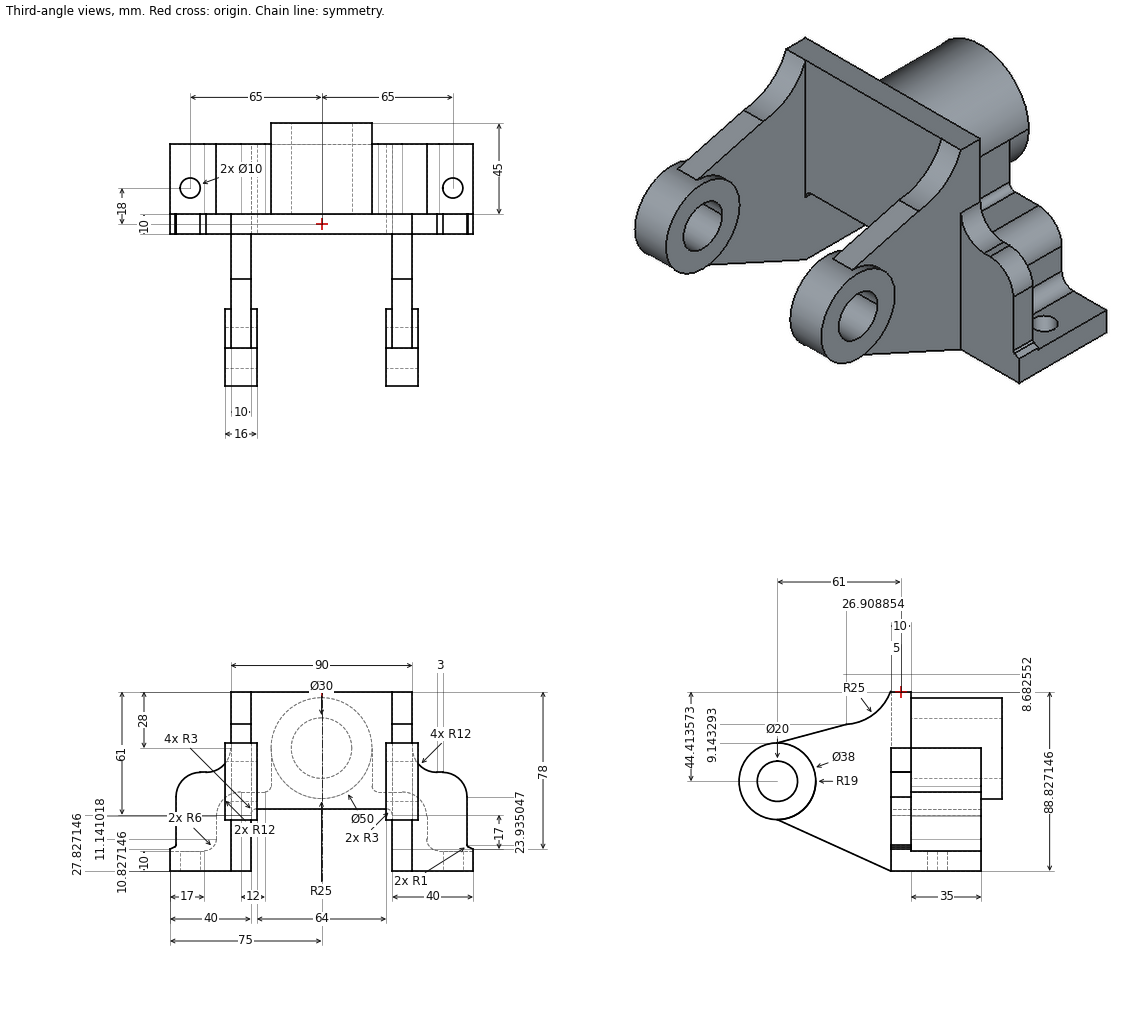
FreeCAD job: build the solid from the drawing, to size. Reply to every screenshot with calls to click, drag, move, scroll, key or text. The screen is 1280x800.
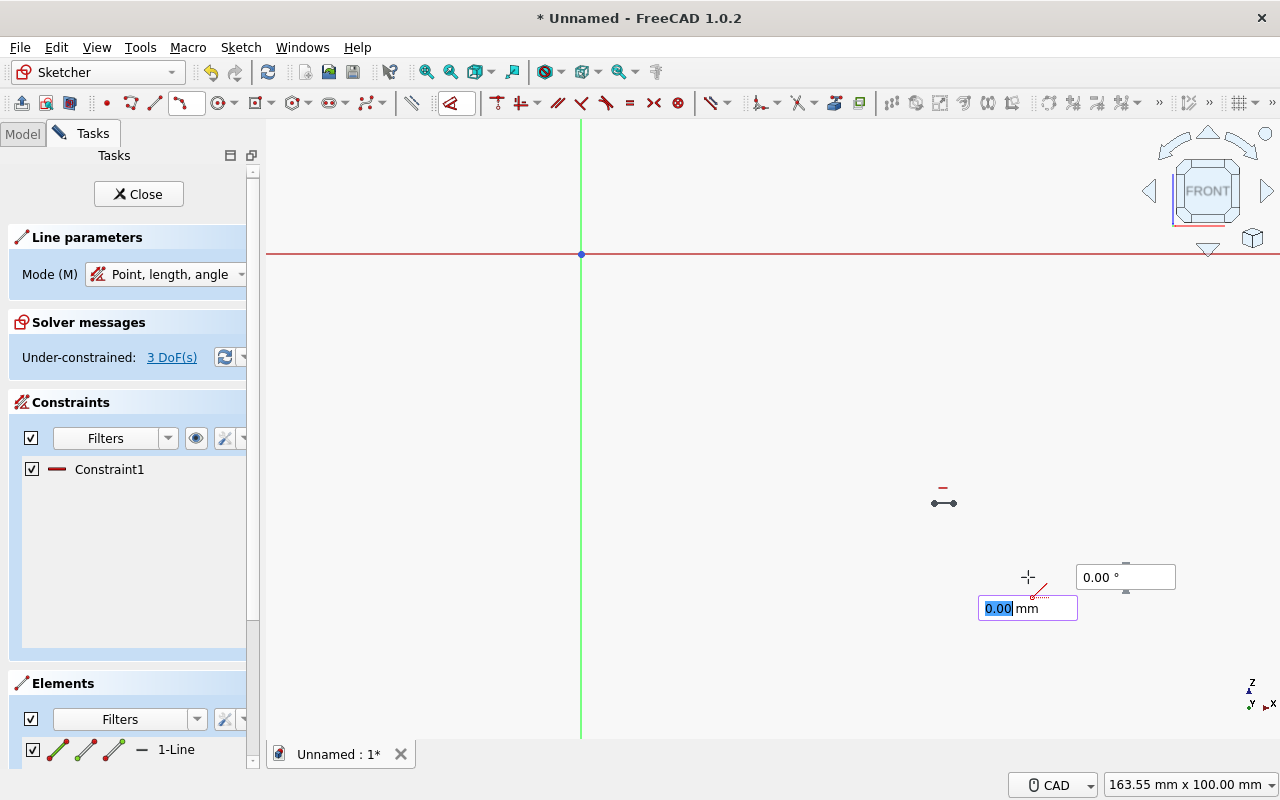
scroll(955, 293, down, 2)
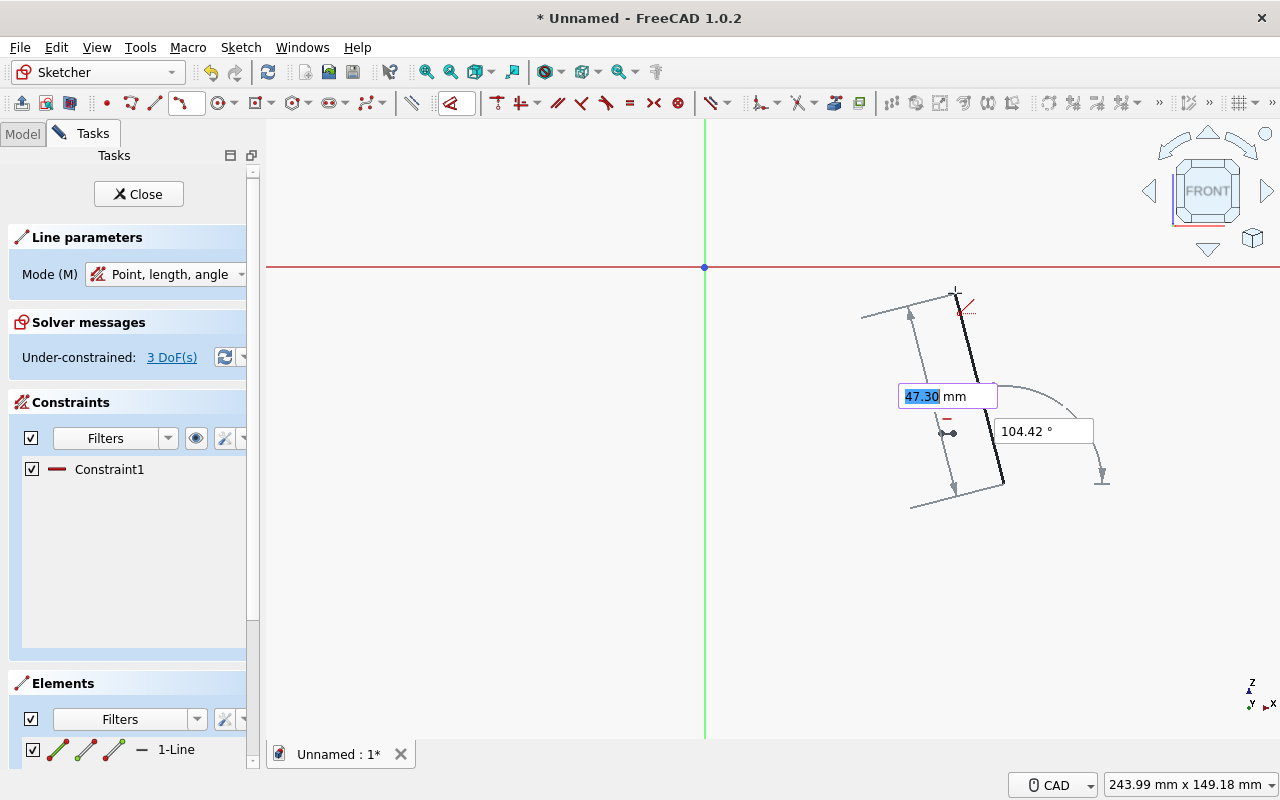
click(1004, 583)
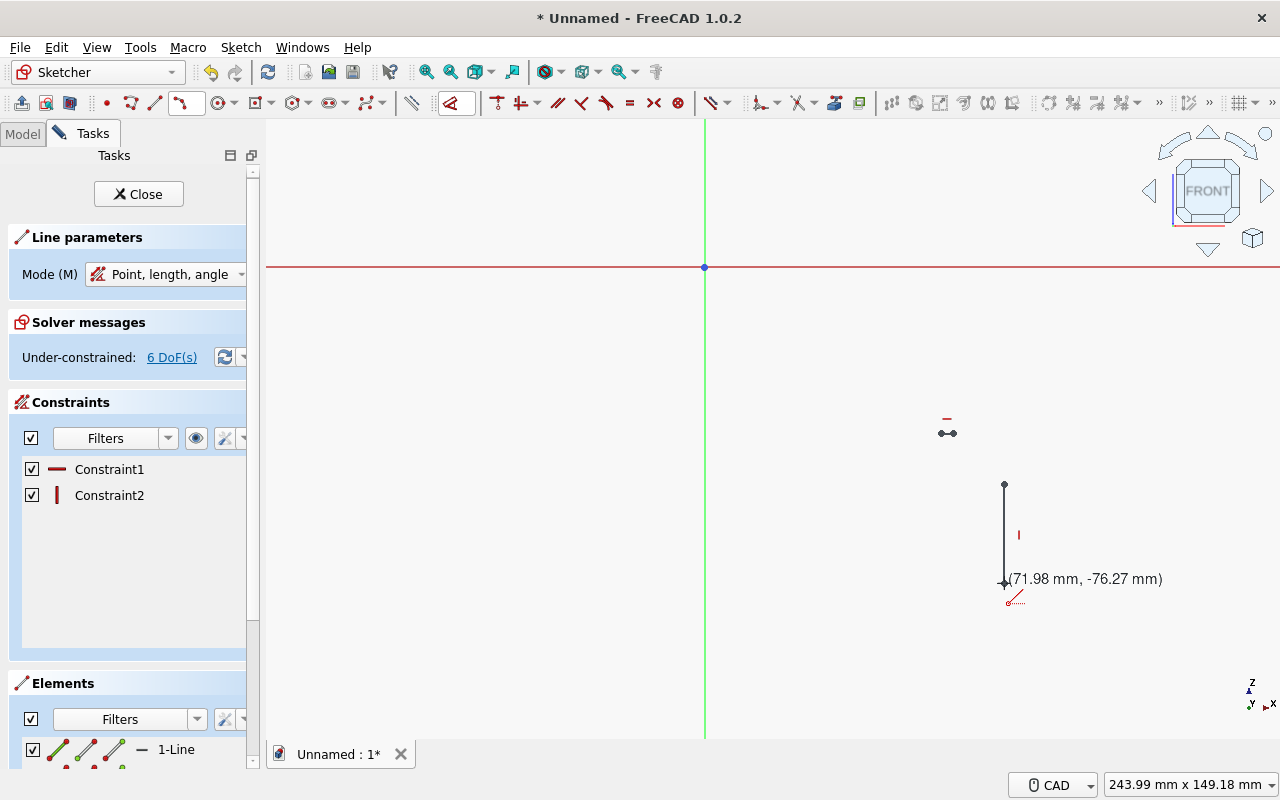
key(g)
key(m)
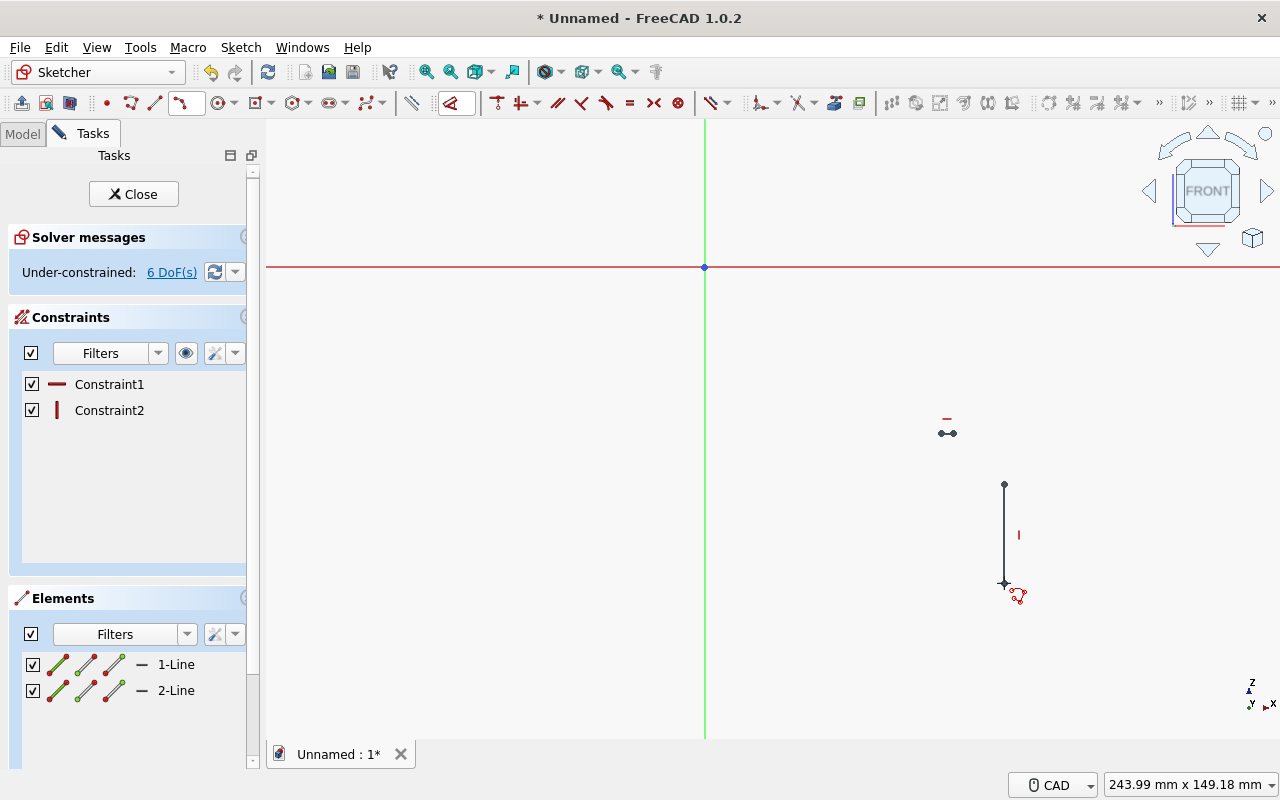
scroll(1006, 586, up, 7)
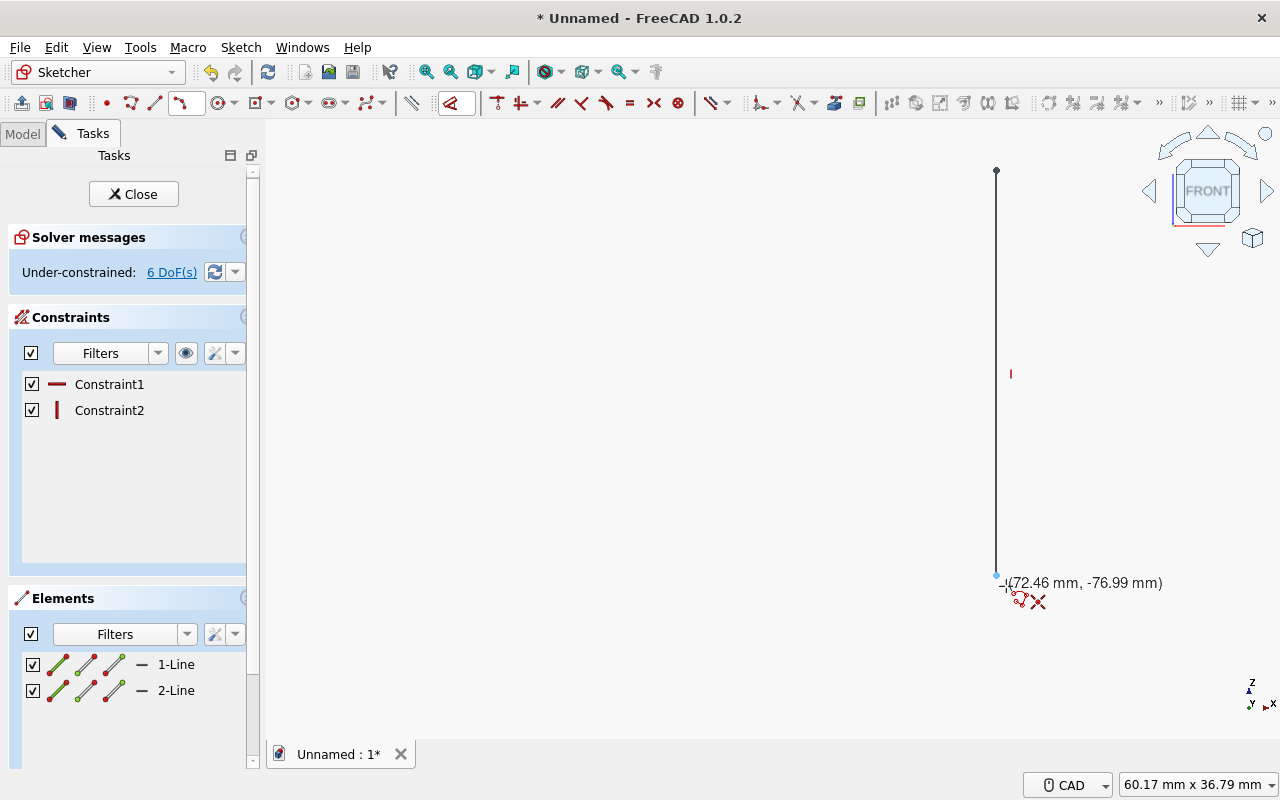
click(1006, 585)
click(1047, 605)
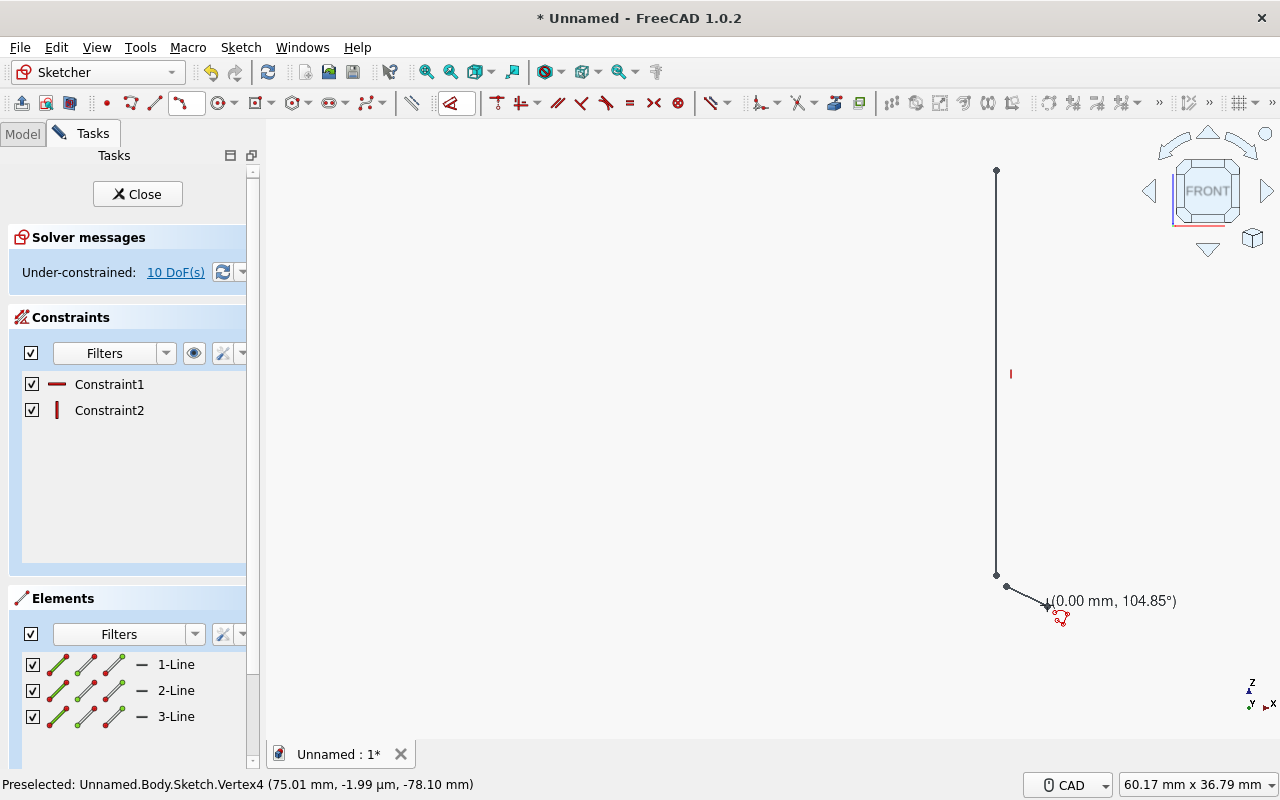
scroll(1006, 587, down, 7)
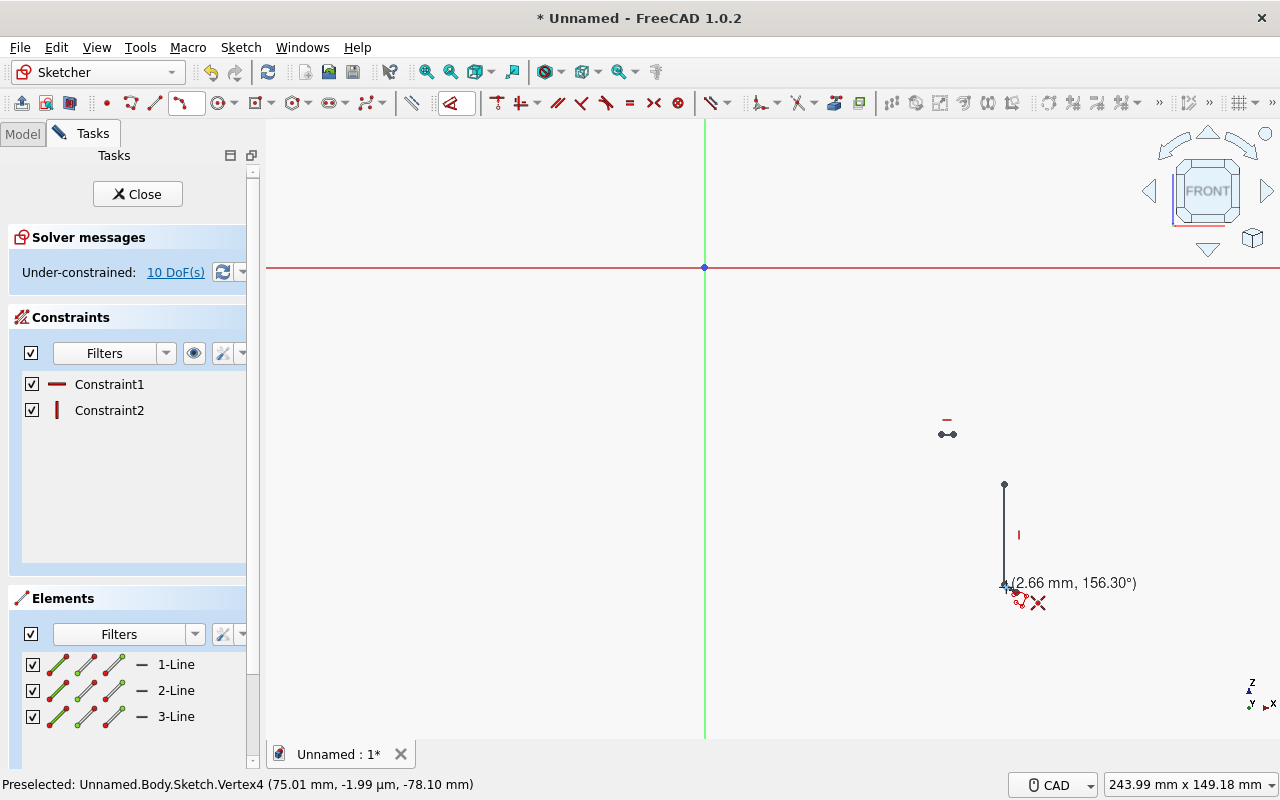
click(850, 592)
click(850, 521)
right_click(850, 521)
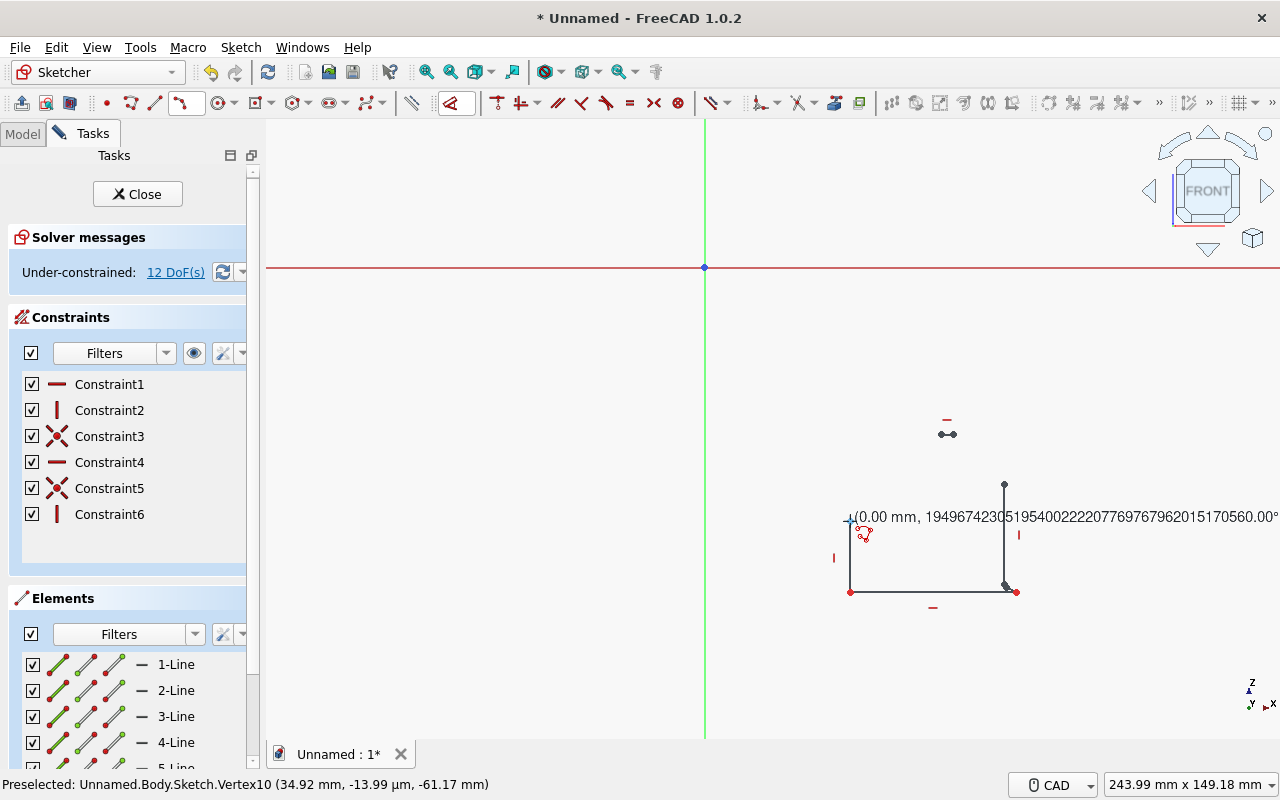
key(g)
key(l)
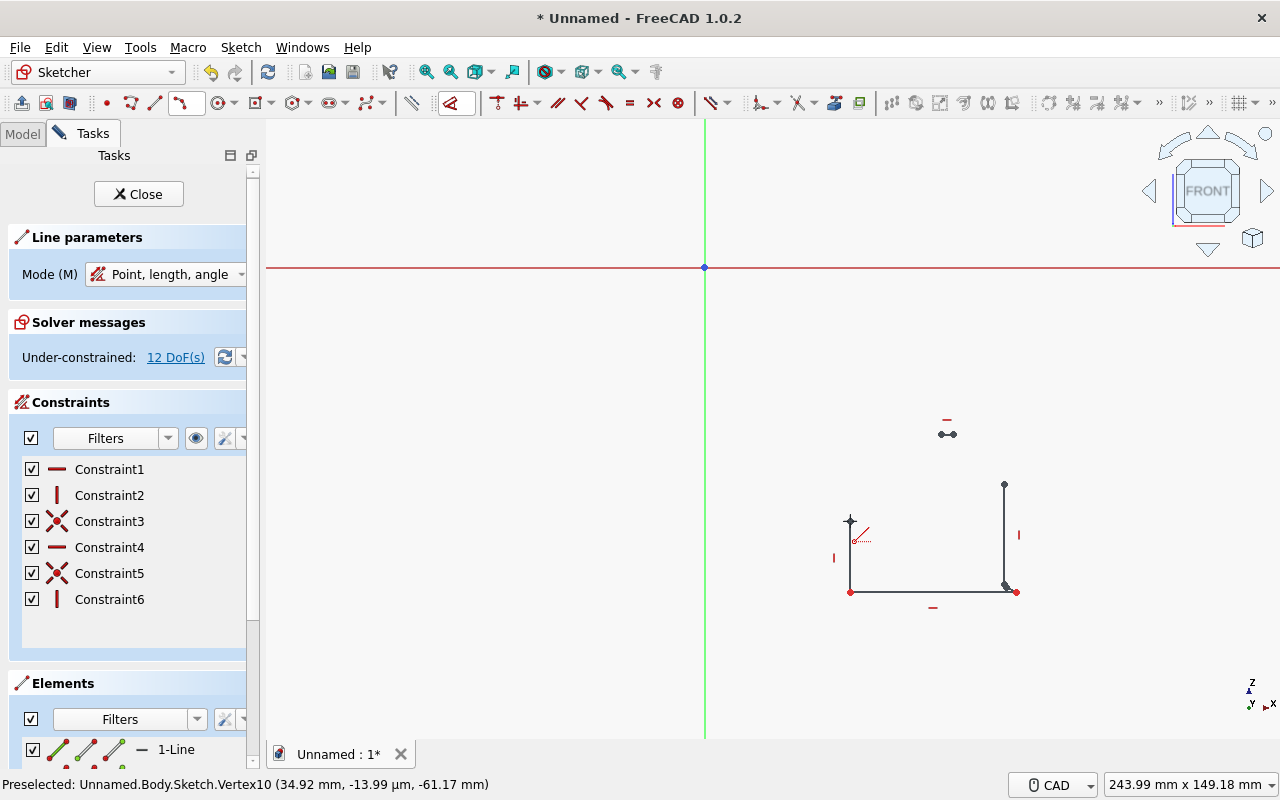
click(838, 509)
click(572, 509)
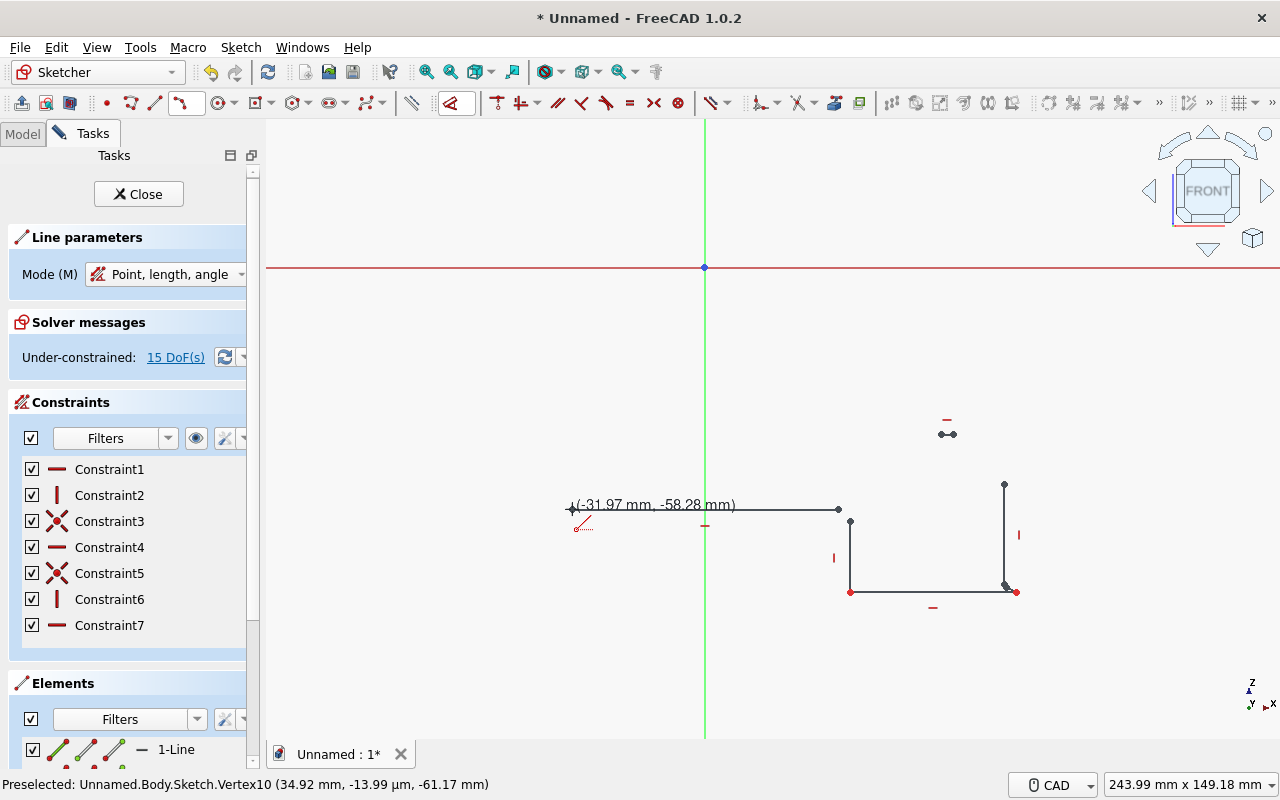
click(132, 104)